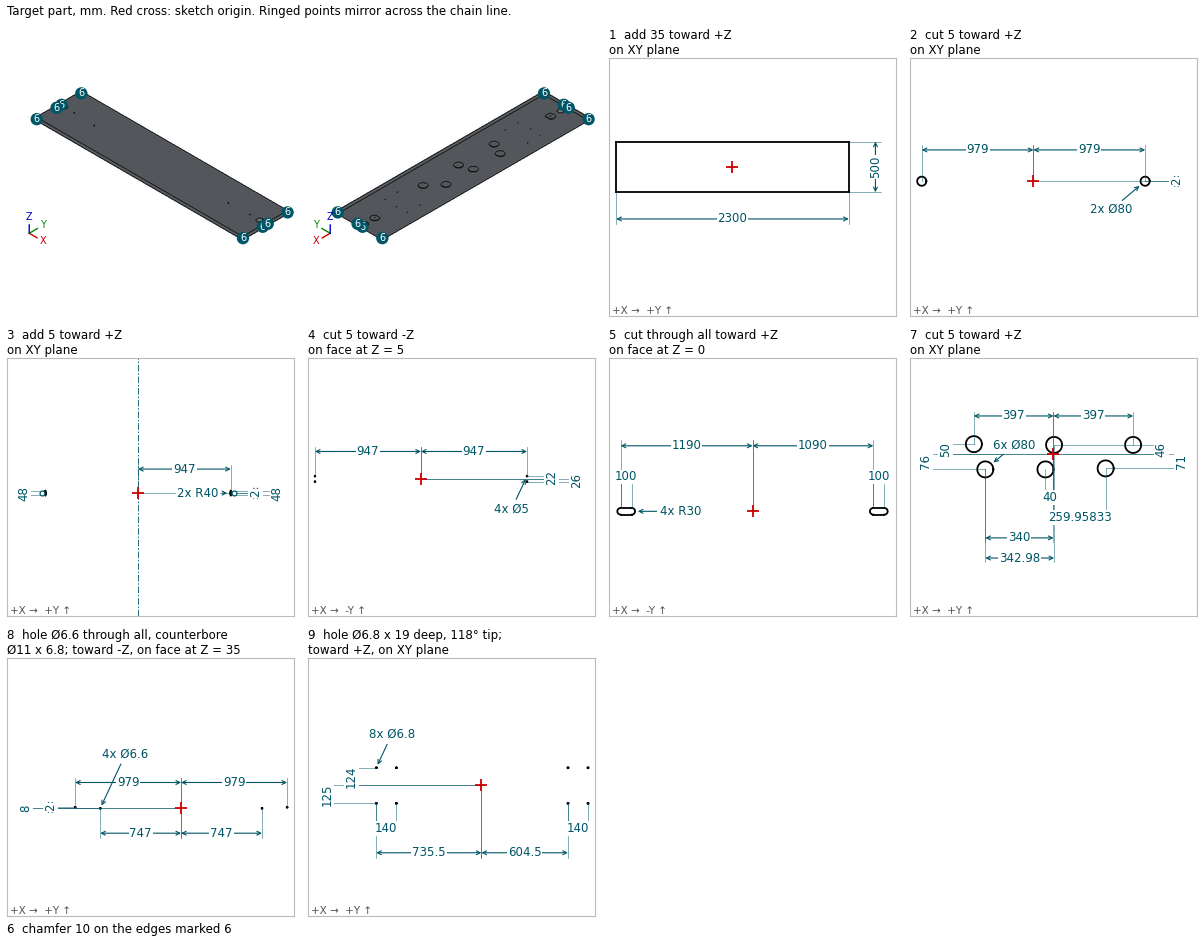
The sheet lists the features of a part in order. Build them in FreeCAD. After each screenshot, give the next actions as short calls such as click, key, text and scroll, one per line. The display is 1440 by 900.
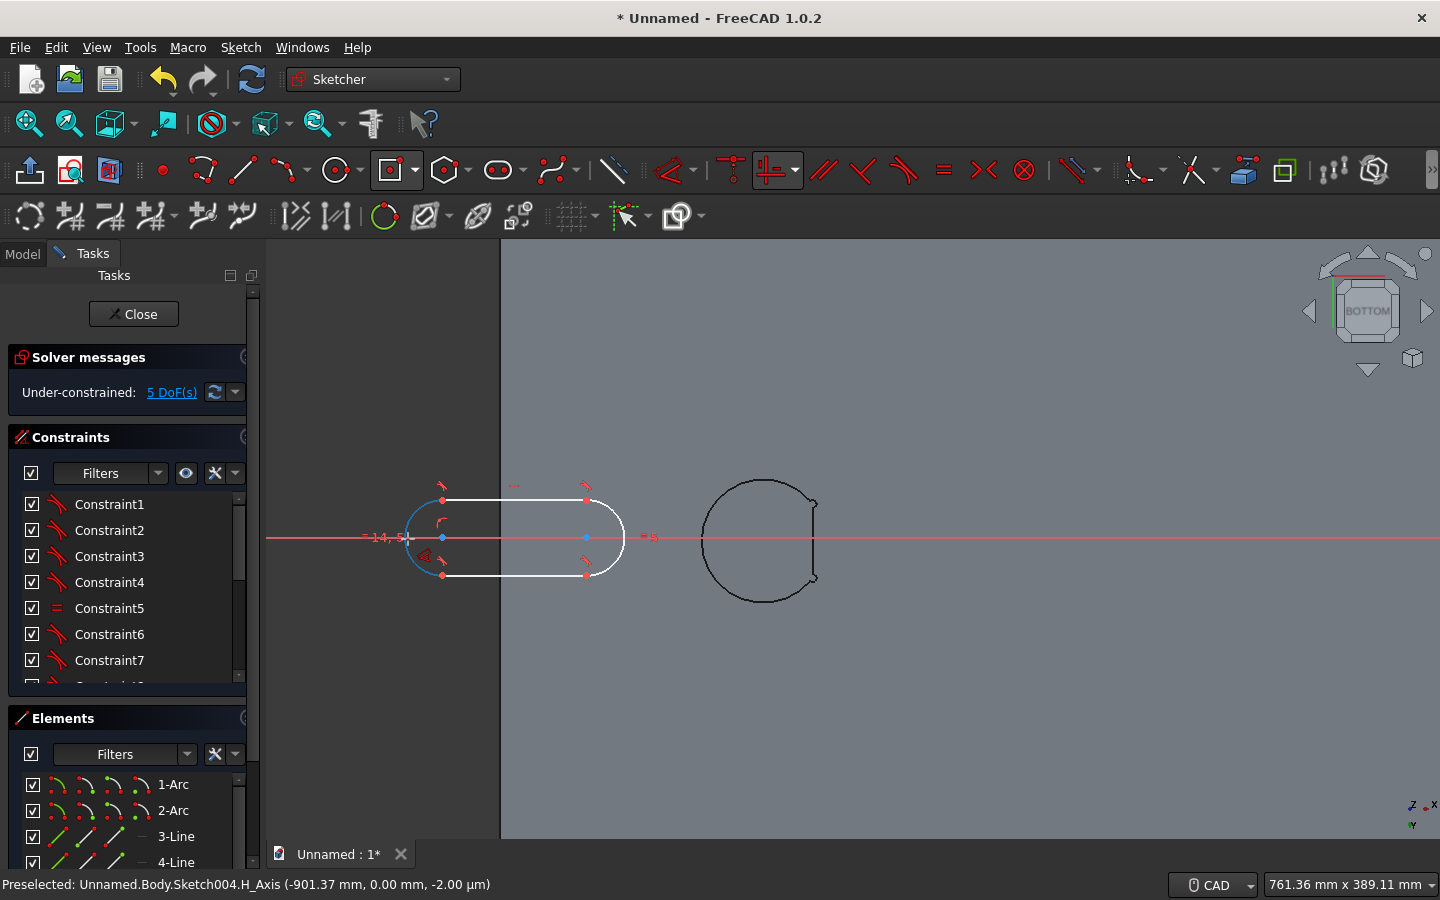
click(405, 538)
click(382, 504)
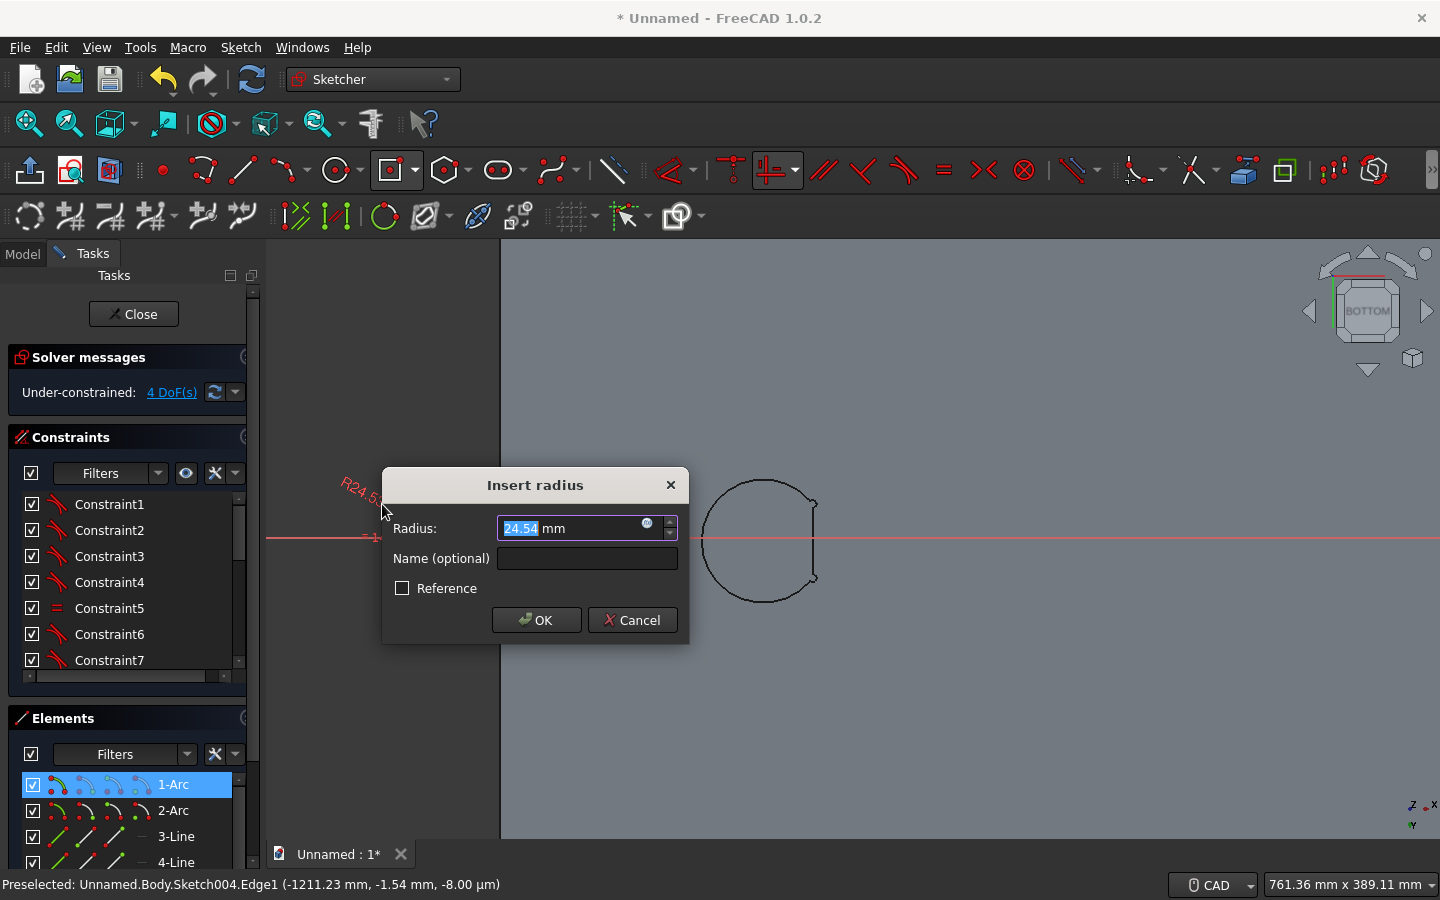
text(30)
key(Return)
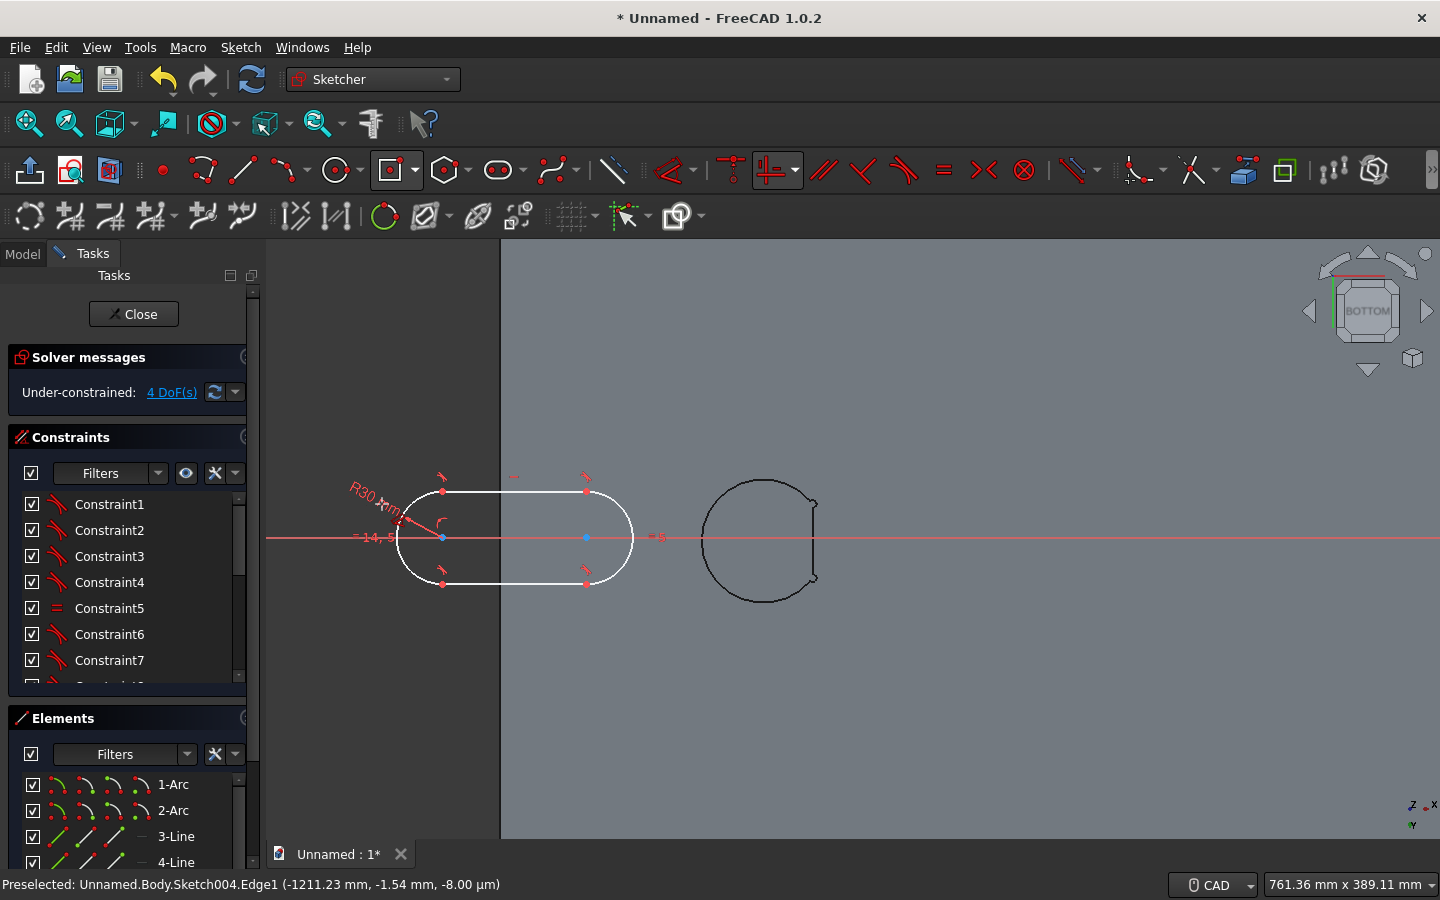
scroll(408, 539, down, 8)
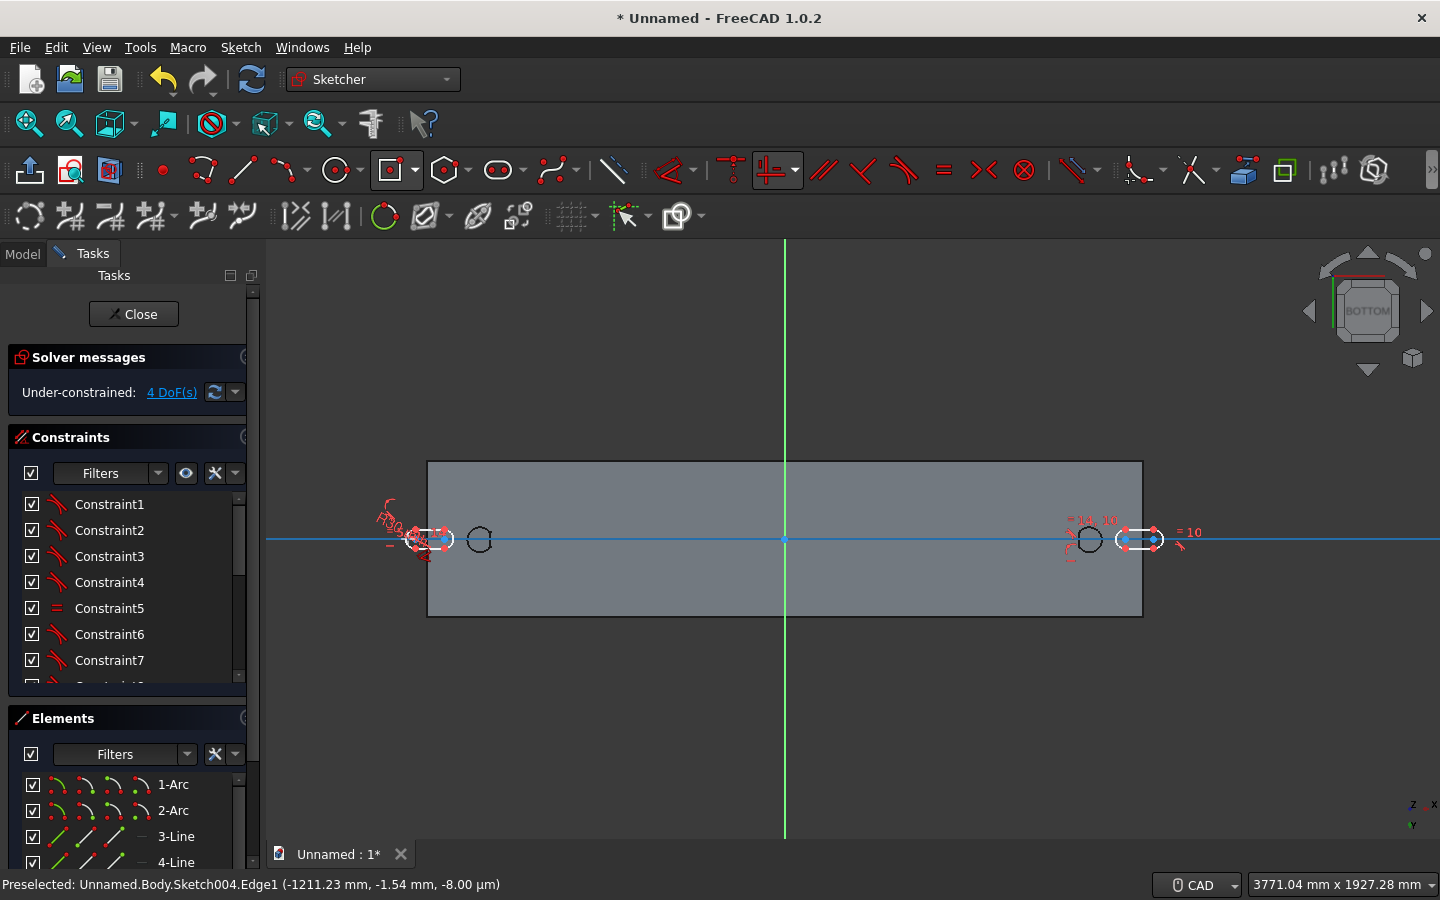
scroll(424, 530, up, 3)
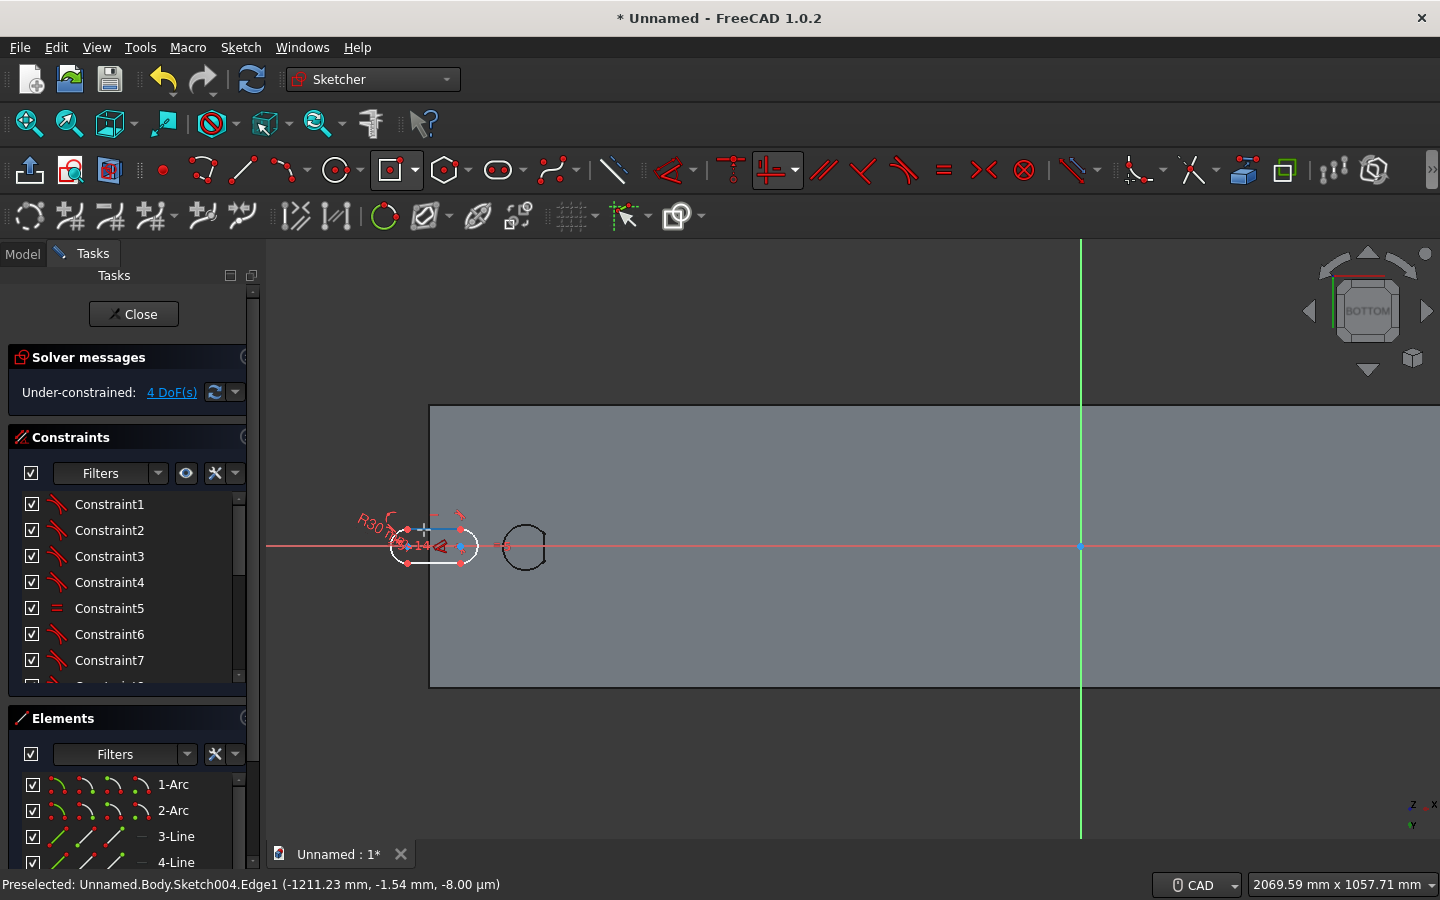
click(424, 529)
click(434, 495)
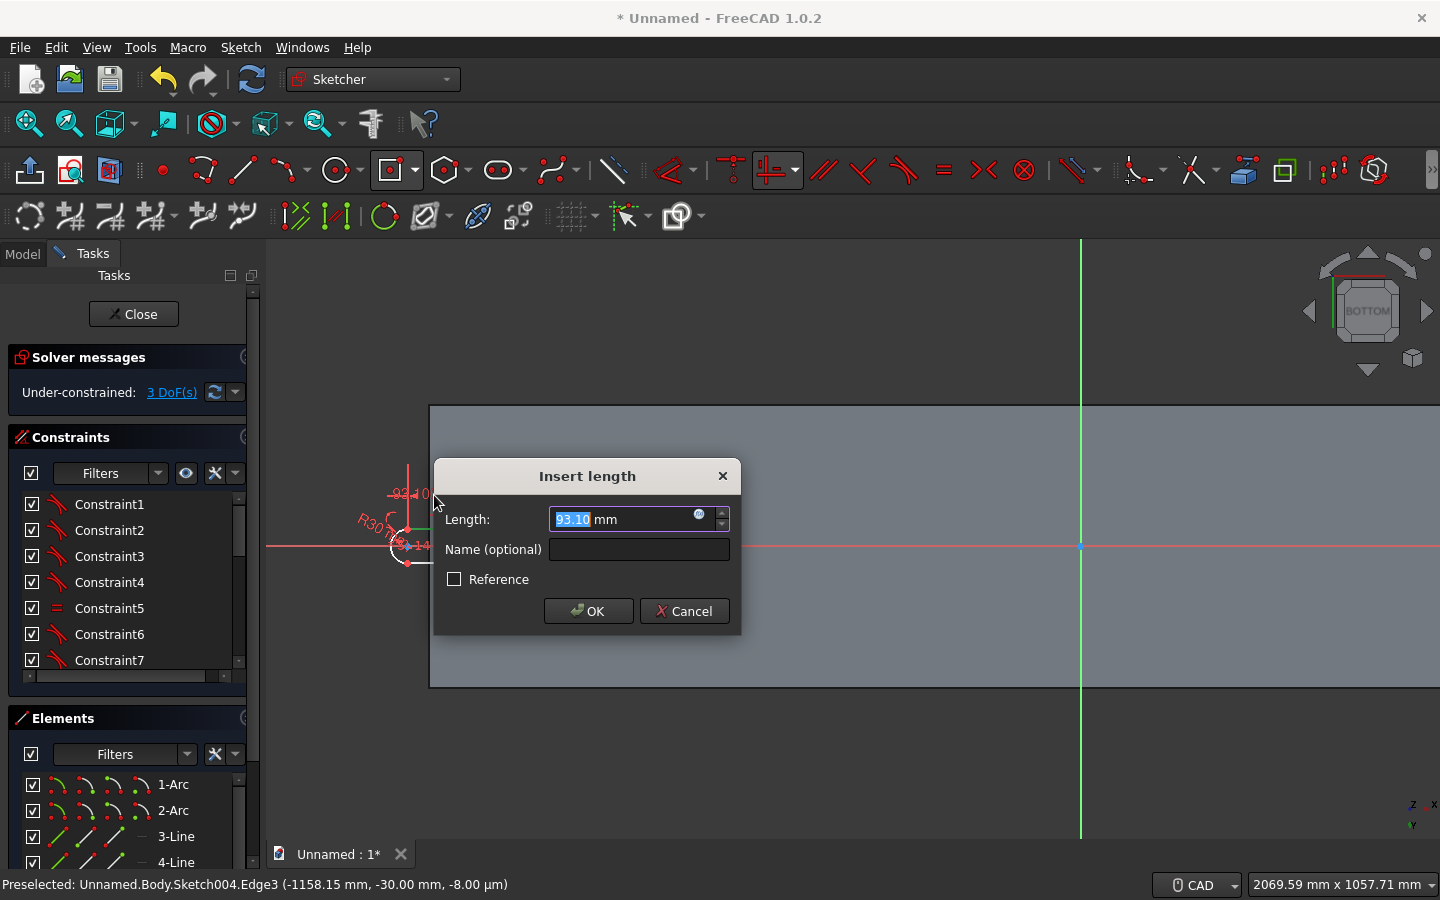
text(100)
key(Return)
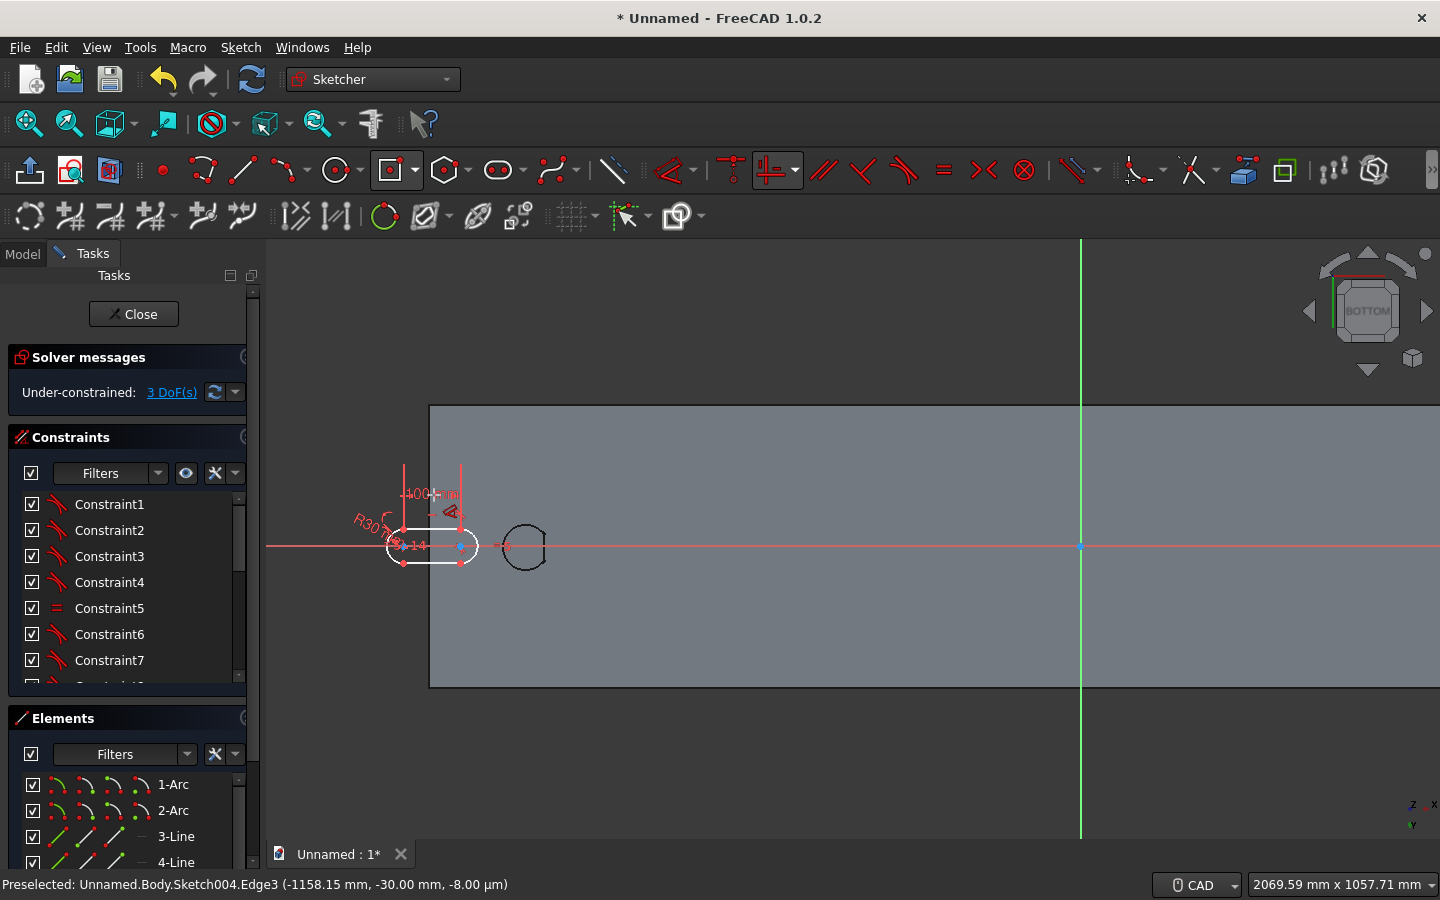
scroll(424, 530, down, 3)